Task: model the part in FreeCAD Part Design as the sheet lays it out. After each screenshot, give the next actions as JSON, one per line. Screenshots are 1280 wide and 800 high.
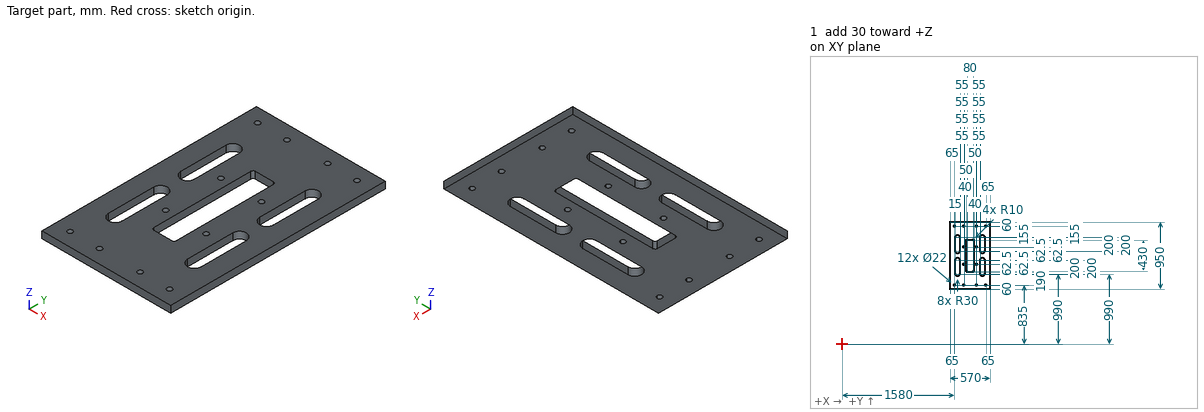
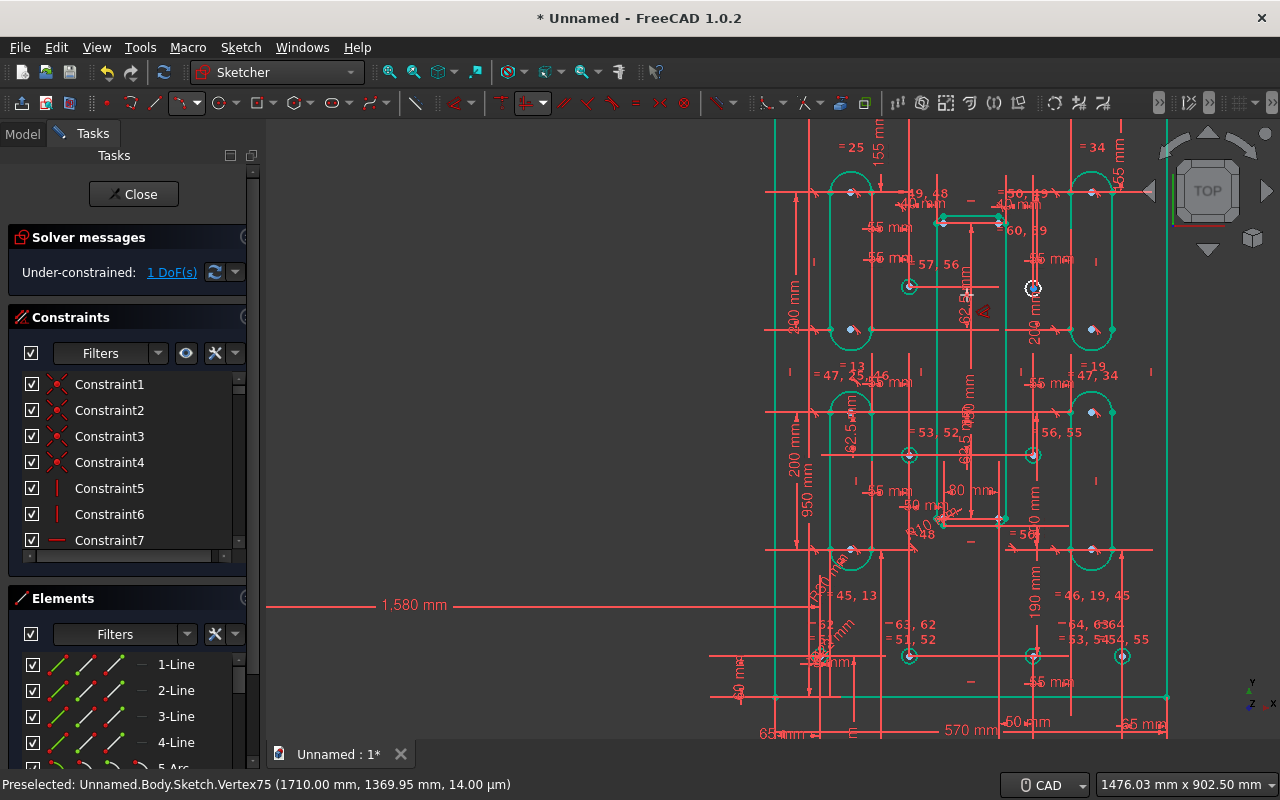
{"action": "left_click", "coordinate": [1071, 330]}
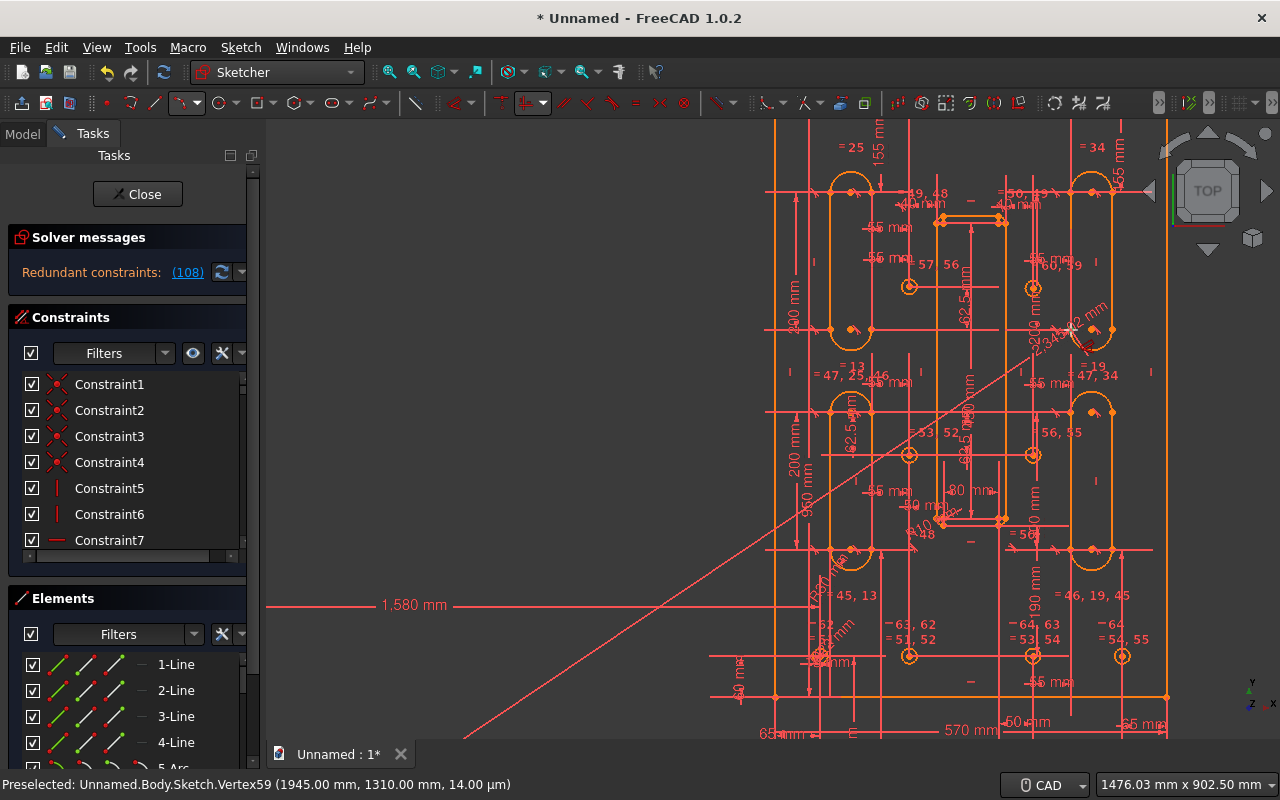
{"action": "left_click", "coordinate": [1033, 288]}
{"action": "left_click", "coordinate": [951, 319]}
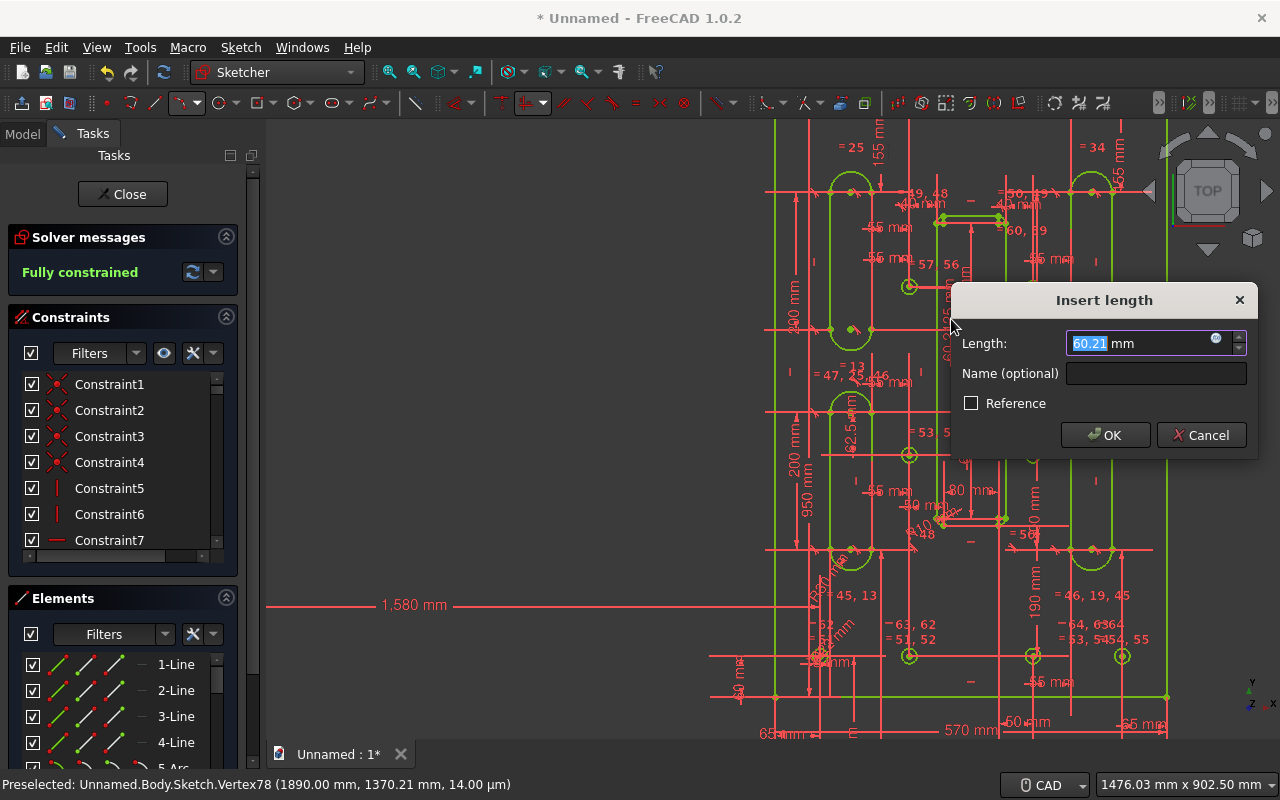
{"action": "type", "text": "62.5"}
{"action": "key", "text": "Return"}
{"action": "key", "text": "Escape"}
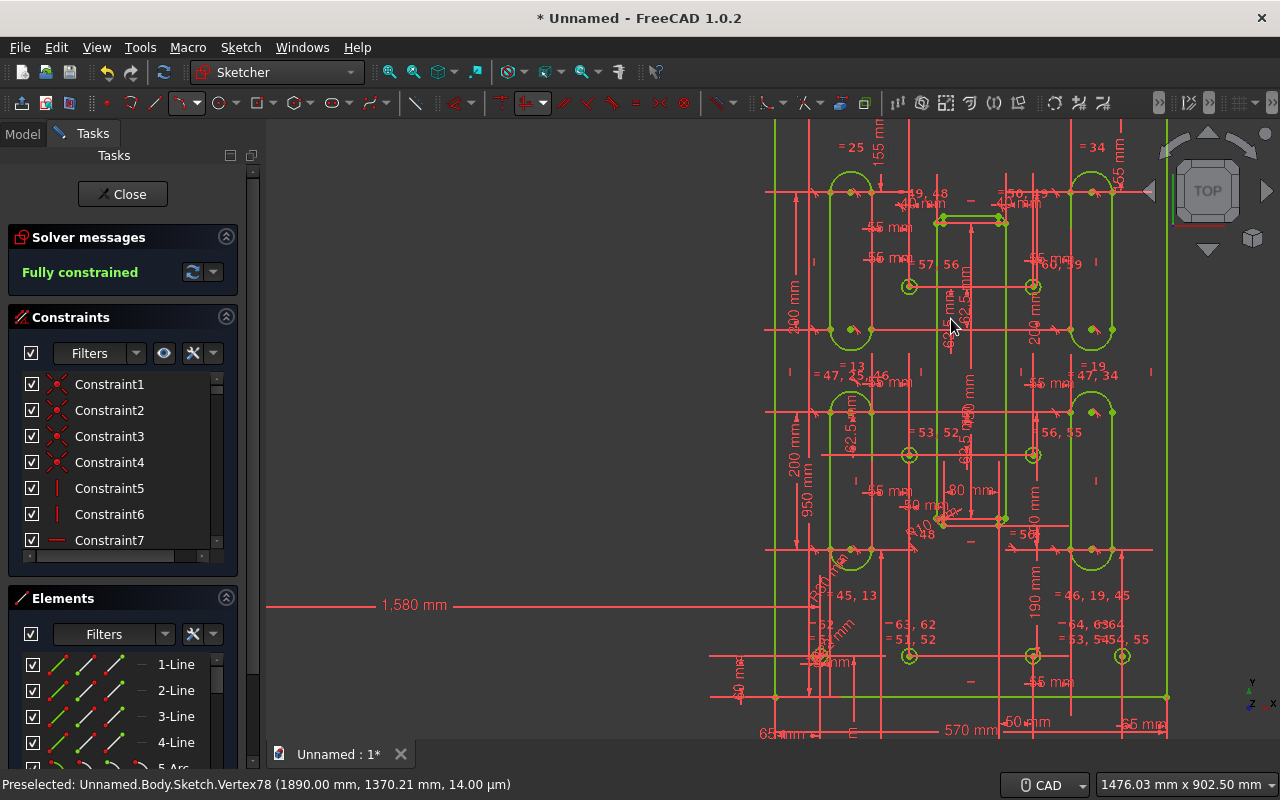
{"action": "left_click", "coordinate": [123, 194]}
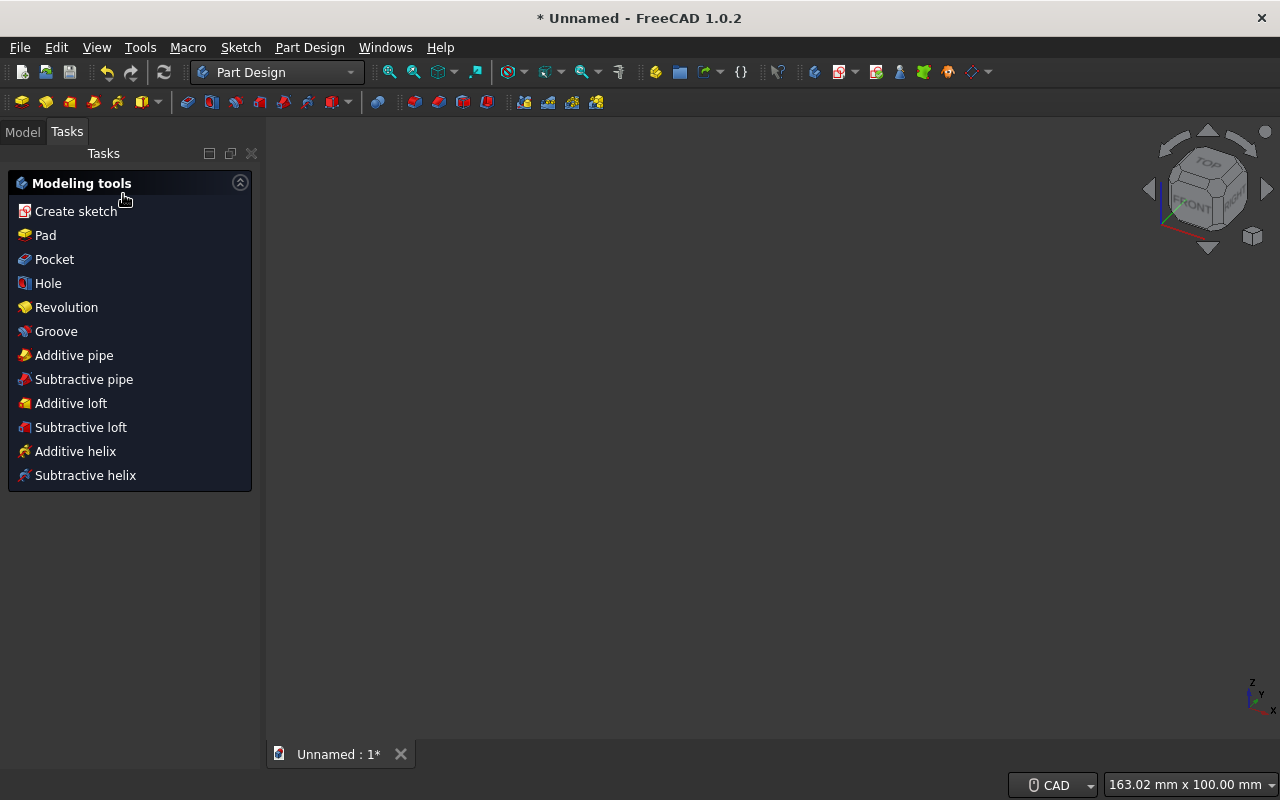
{"action": "left_click", "coordinate": [22, 102]}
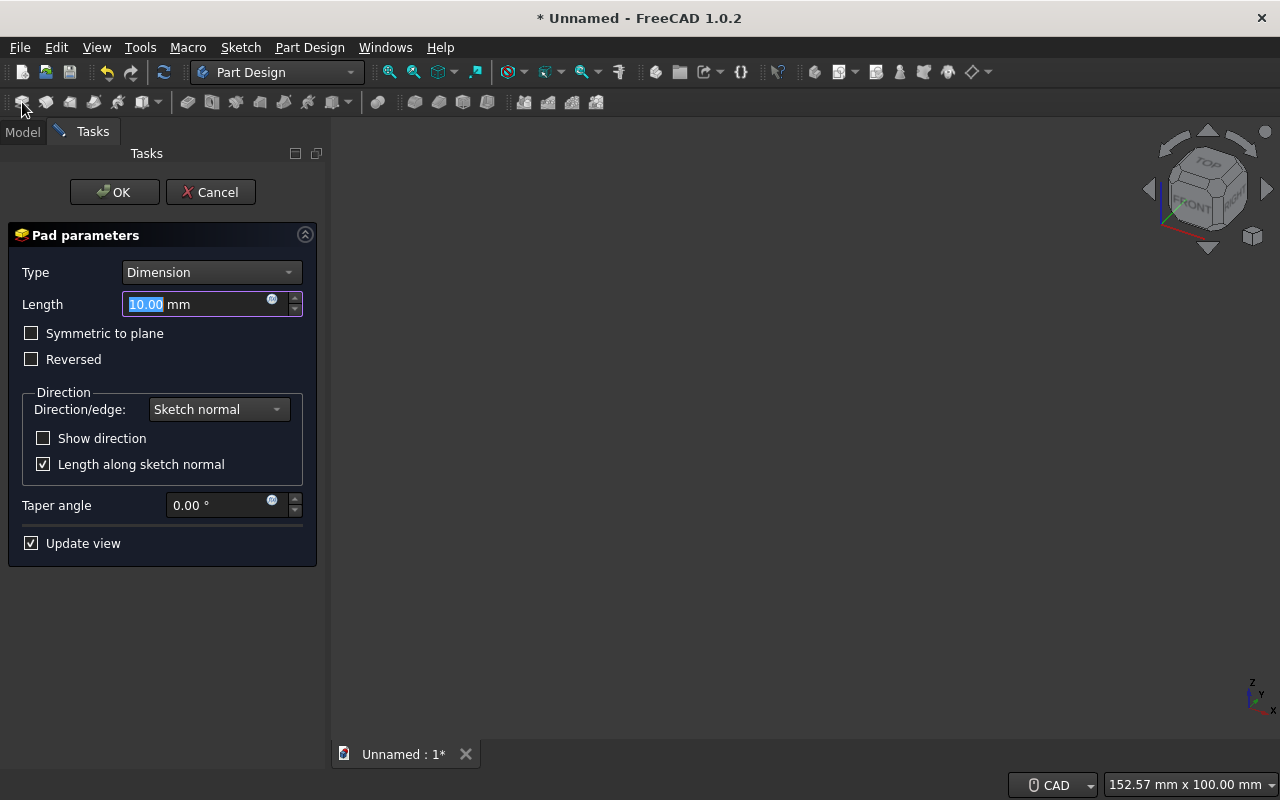
{"action": "type", "text": "30"}
{"action": "key", "text": "Tab"}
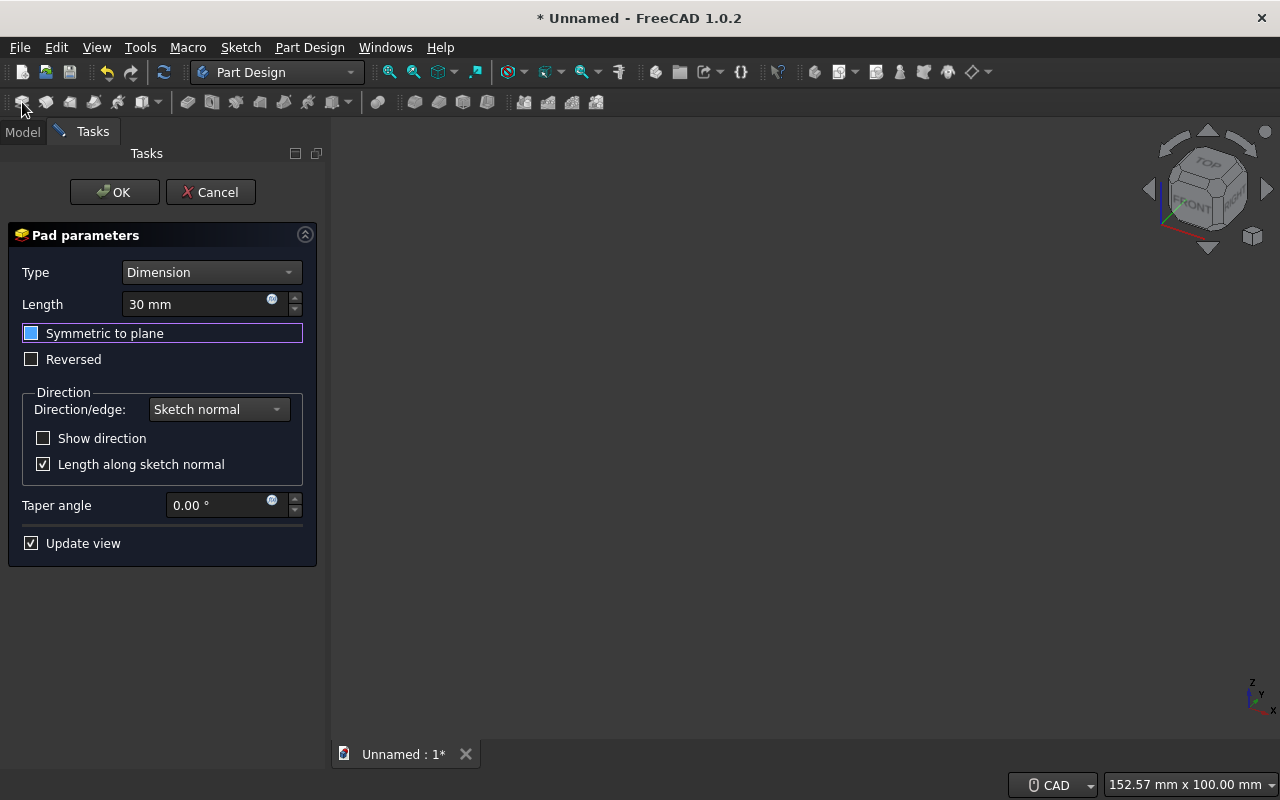
{"action": "left_click", "coordinate": [115, 192]}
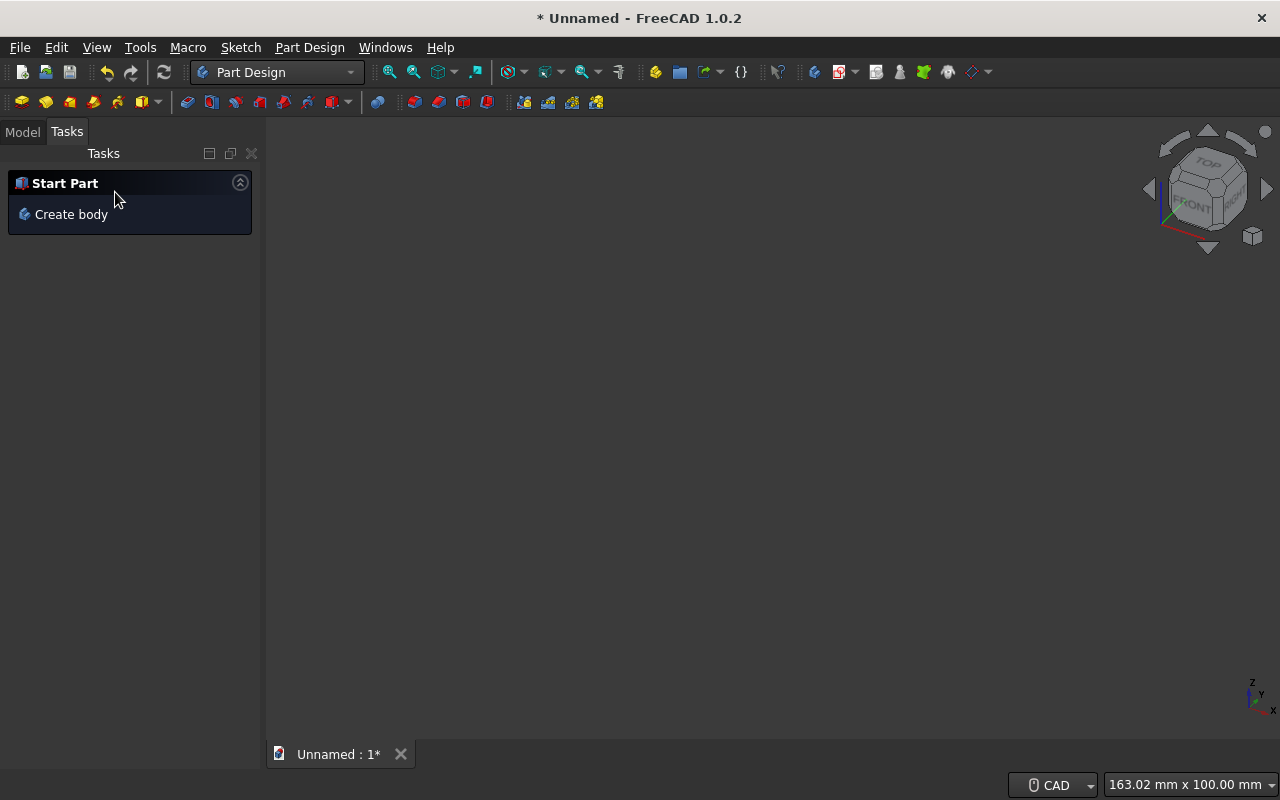
{"action": "key", "text": "0"}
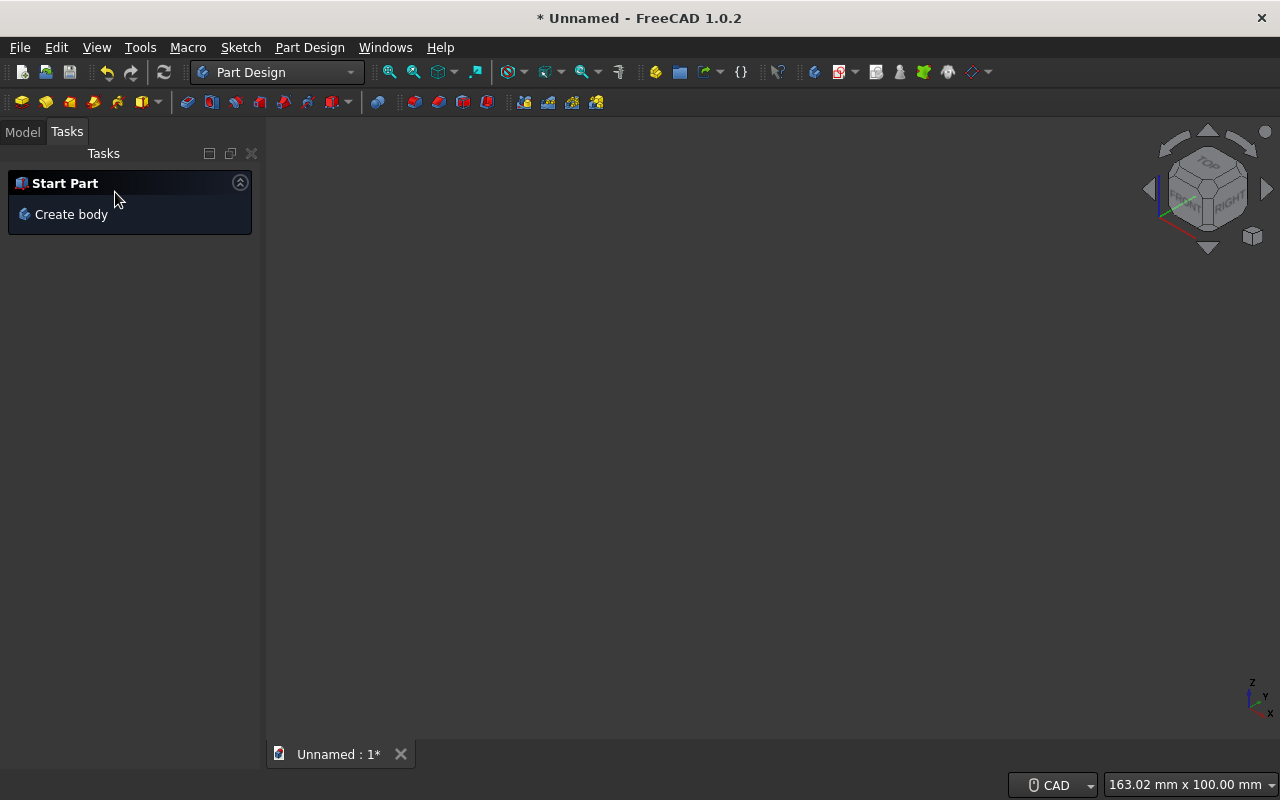
{"action": "left_click", "coordinate": [390, 72]}